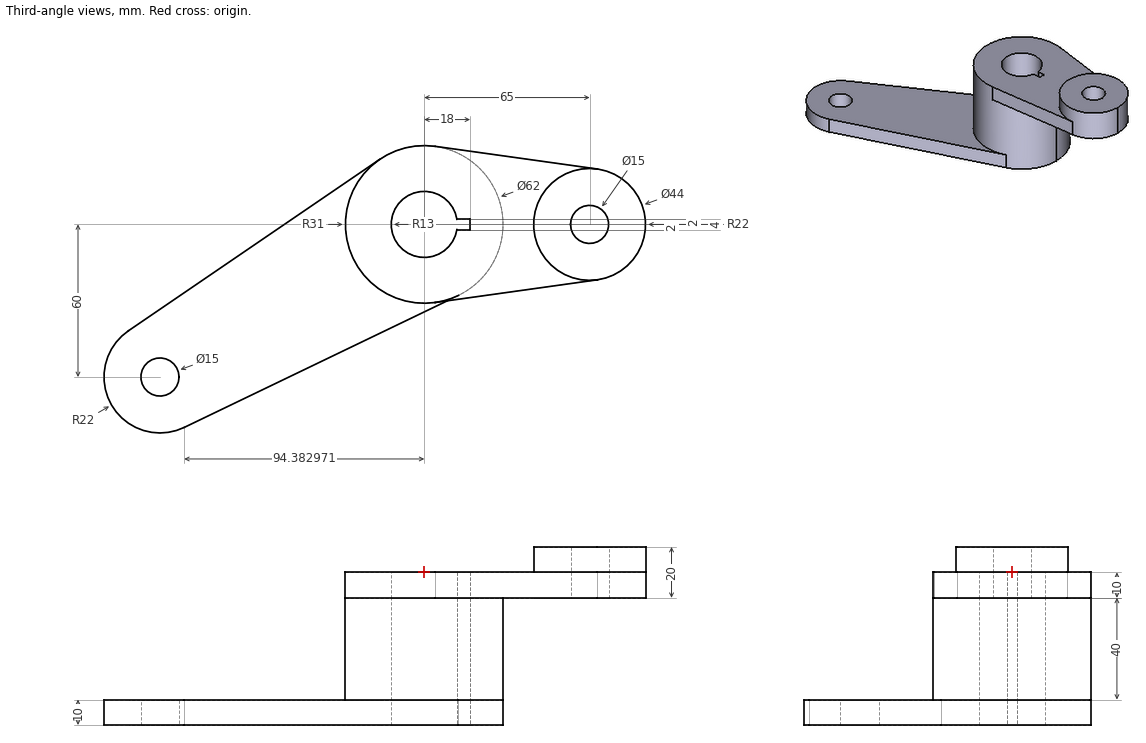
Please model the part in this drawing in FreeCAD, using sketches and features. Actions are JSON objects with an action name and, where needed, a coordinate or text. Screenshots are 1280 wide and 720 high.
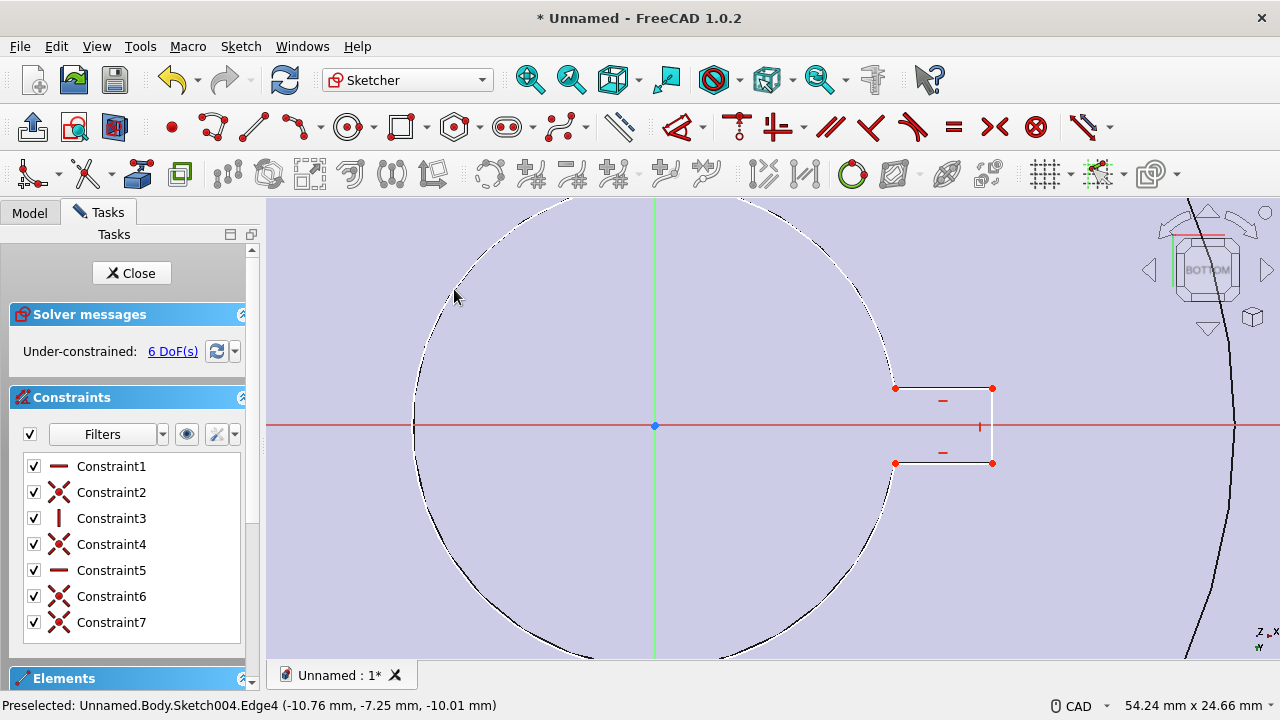
{"action": "left_click_drag", "start_coordinate": [645, 415], "coordinate": [665, 436]}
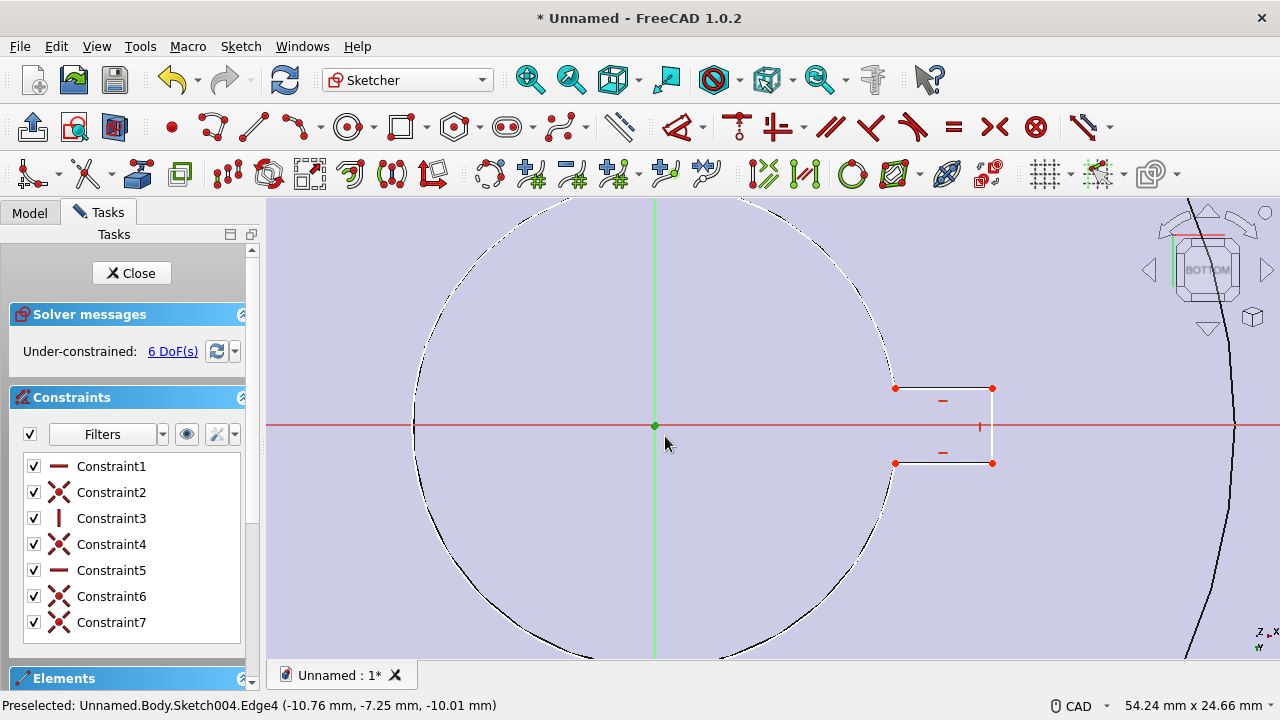
{"action": "key", "text": "c"}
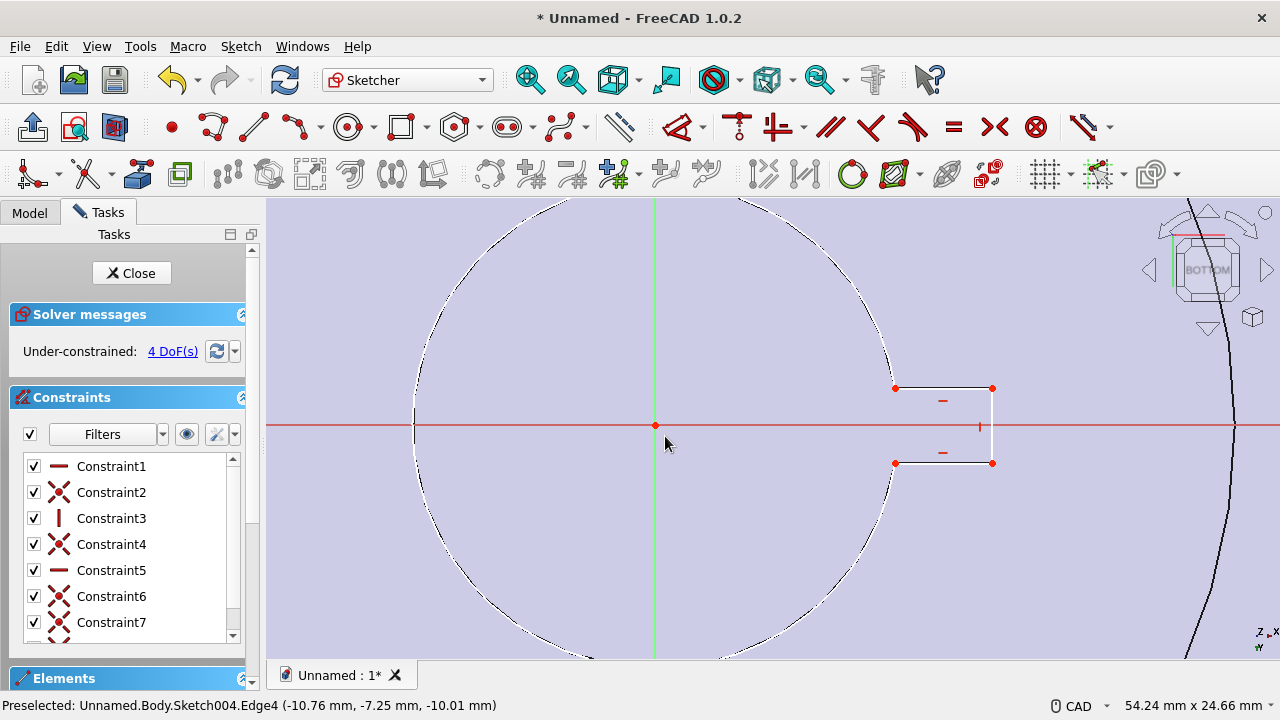
{"action": "key", "text": "d"}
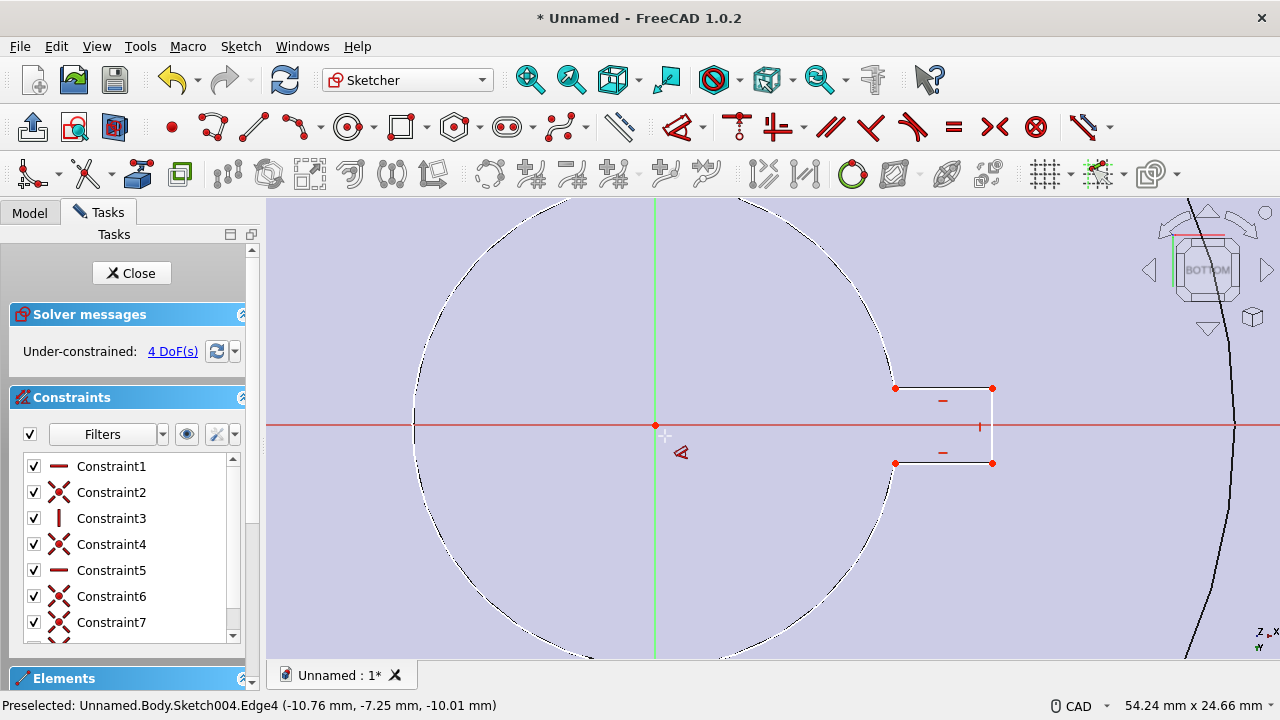
{"action": "left_click", "coordinate": [412, 424]}
{"action": "left_click", "coordinate": [414, 292]}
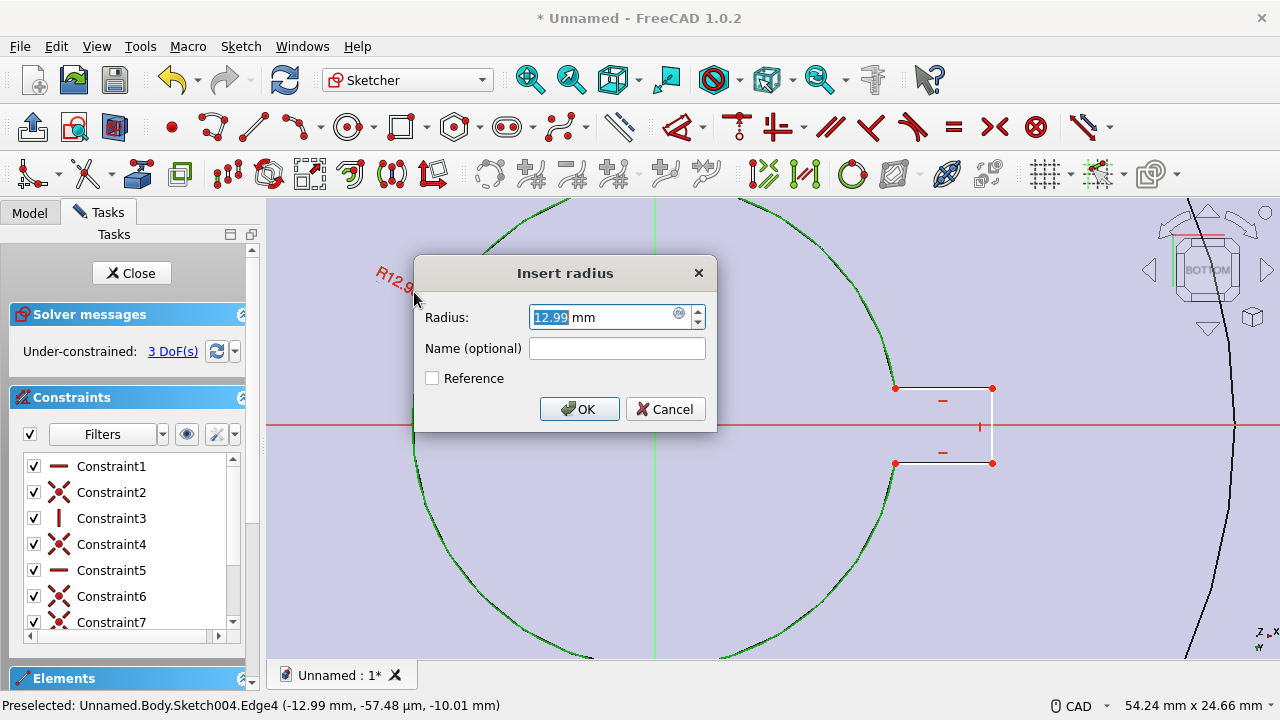
{"action": "type", "text": "13"}
{"action": "key", "text": "Return"}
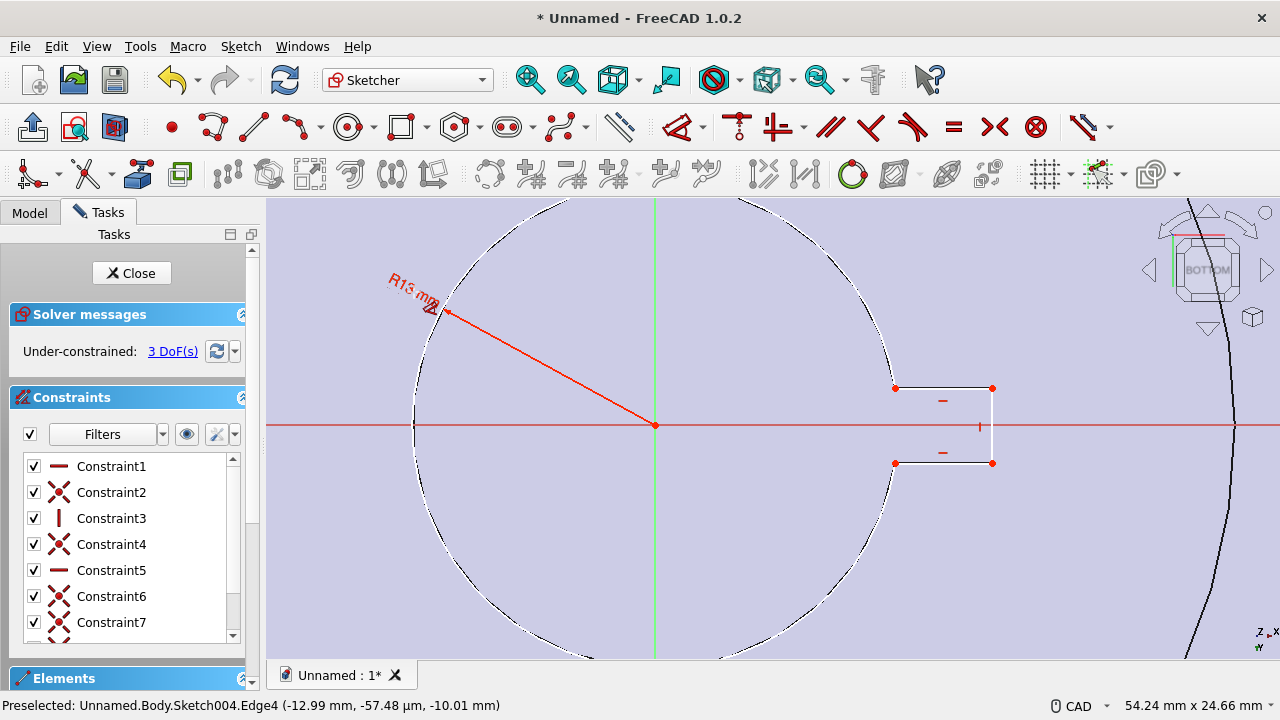
{"action": "left_click", "coordinate": [992, 442]}
{"action": "left_click", "coordinate": [1026, 409]}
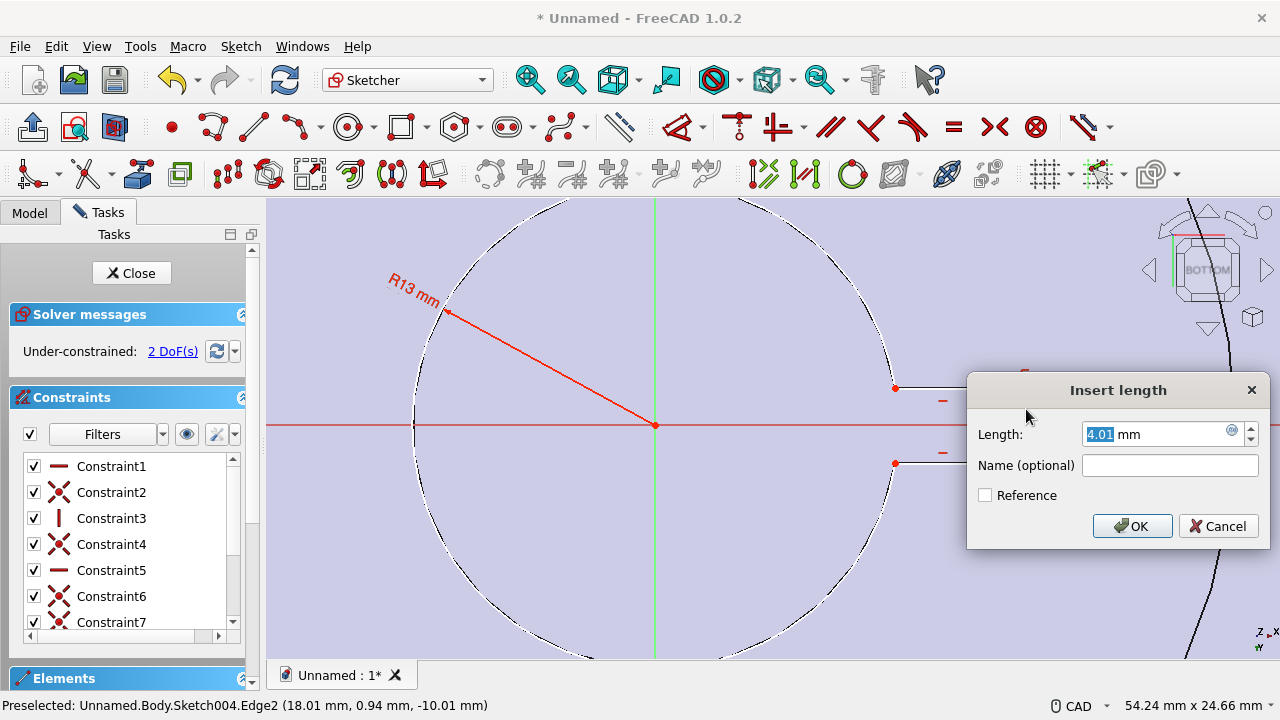
{"action": "type", "text": "4"}
{"action": "key", "text": "Return"}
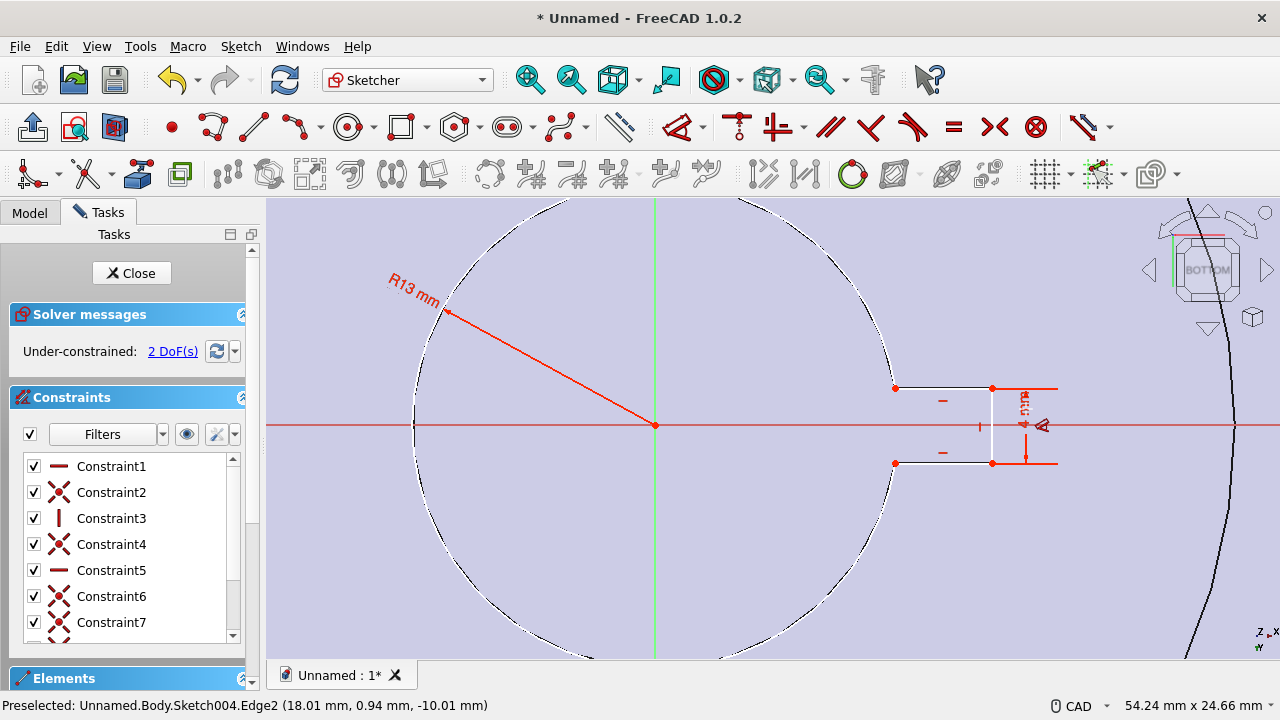
{"action": "left_click", "coordinate": [895, 464]}
{"action": "left_click", "coordinate": [929, 445]}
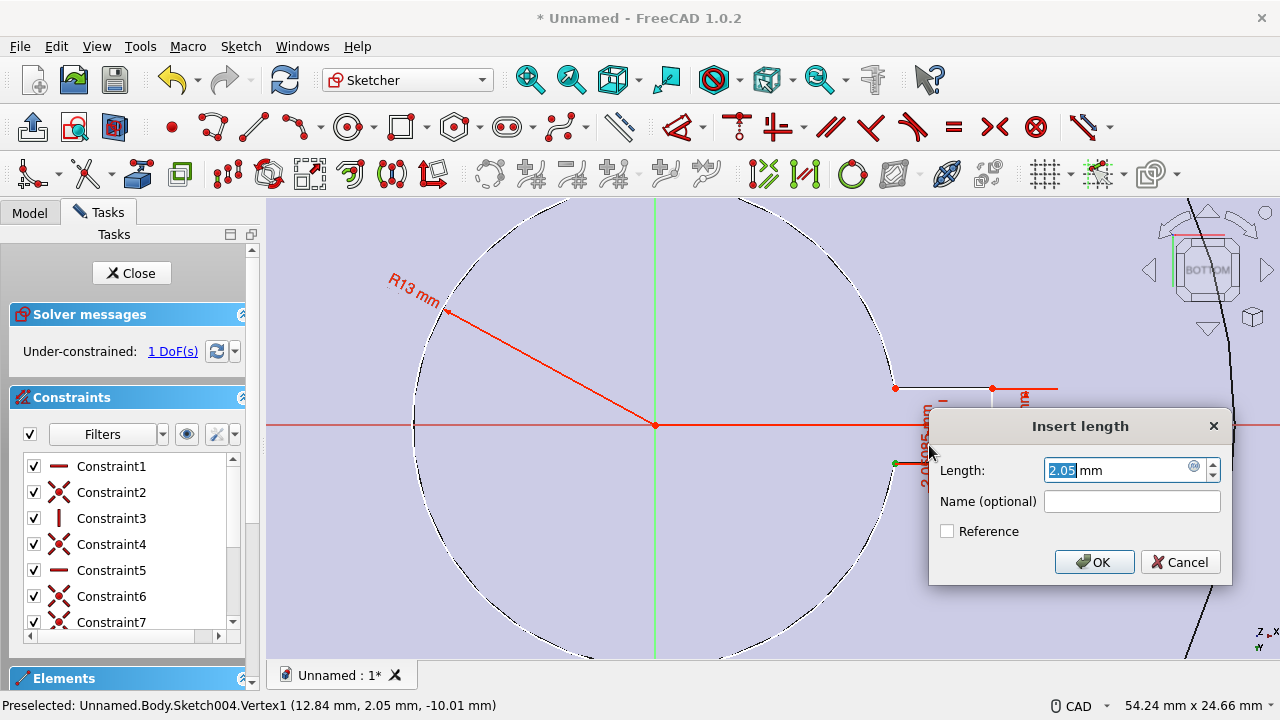
{"action": "type", "text": "2"}
{"action": "key", "text": "Return"}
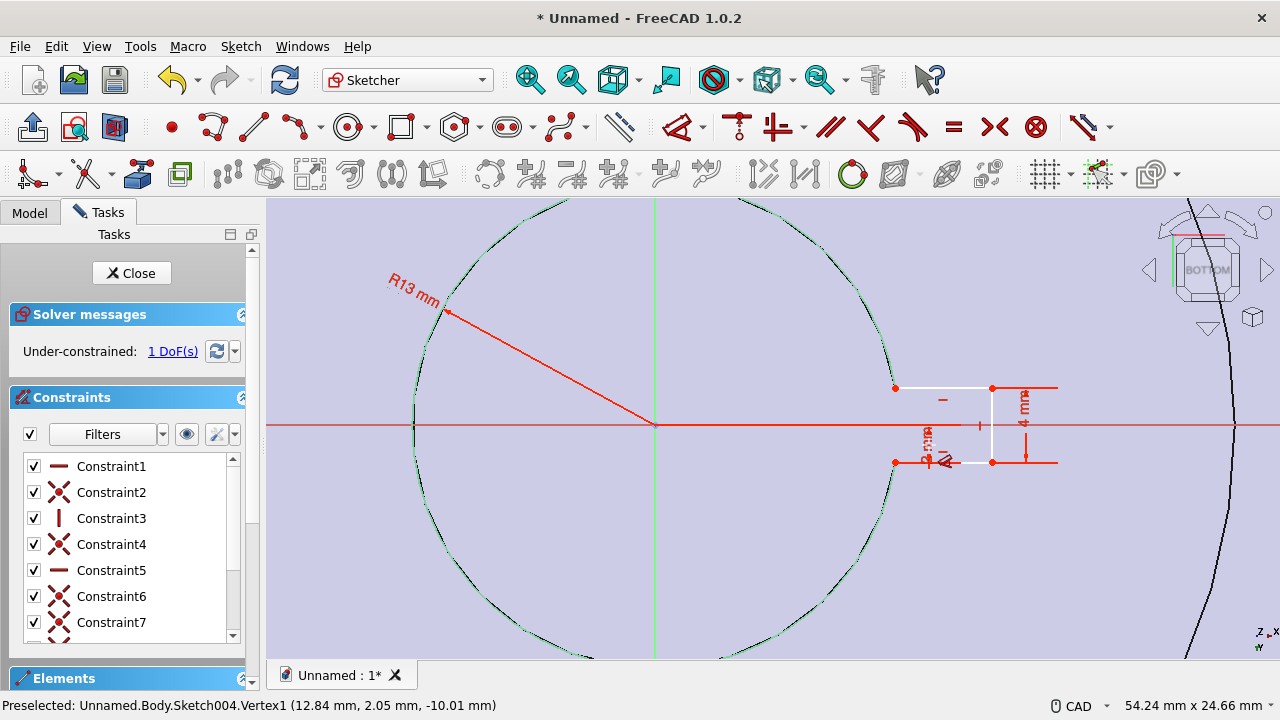
{"action": "left_click", "coordinate": [992, 463]}
{"action": "left_click", "coordinate": [824, 497]}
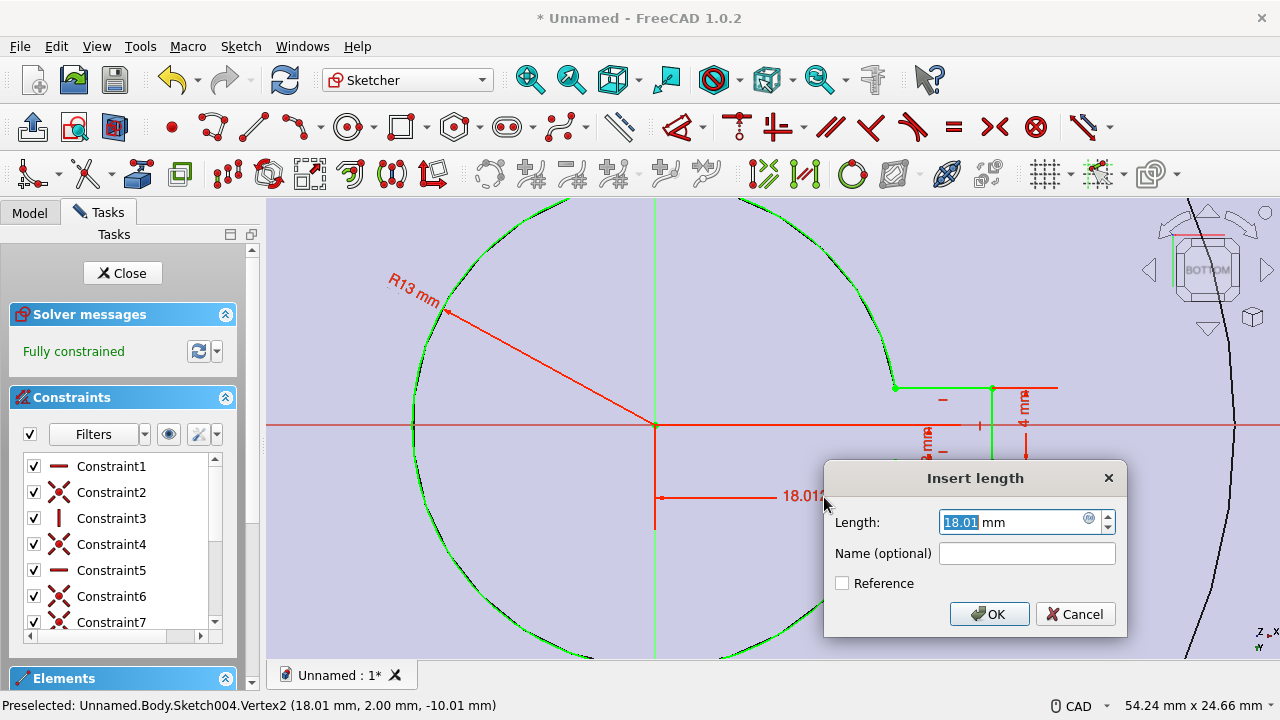
{"action": "type", "text": "18"}
{"action": "key", "text": "Return"}
{"action": "key", "text": "Escape"}